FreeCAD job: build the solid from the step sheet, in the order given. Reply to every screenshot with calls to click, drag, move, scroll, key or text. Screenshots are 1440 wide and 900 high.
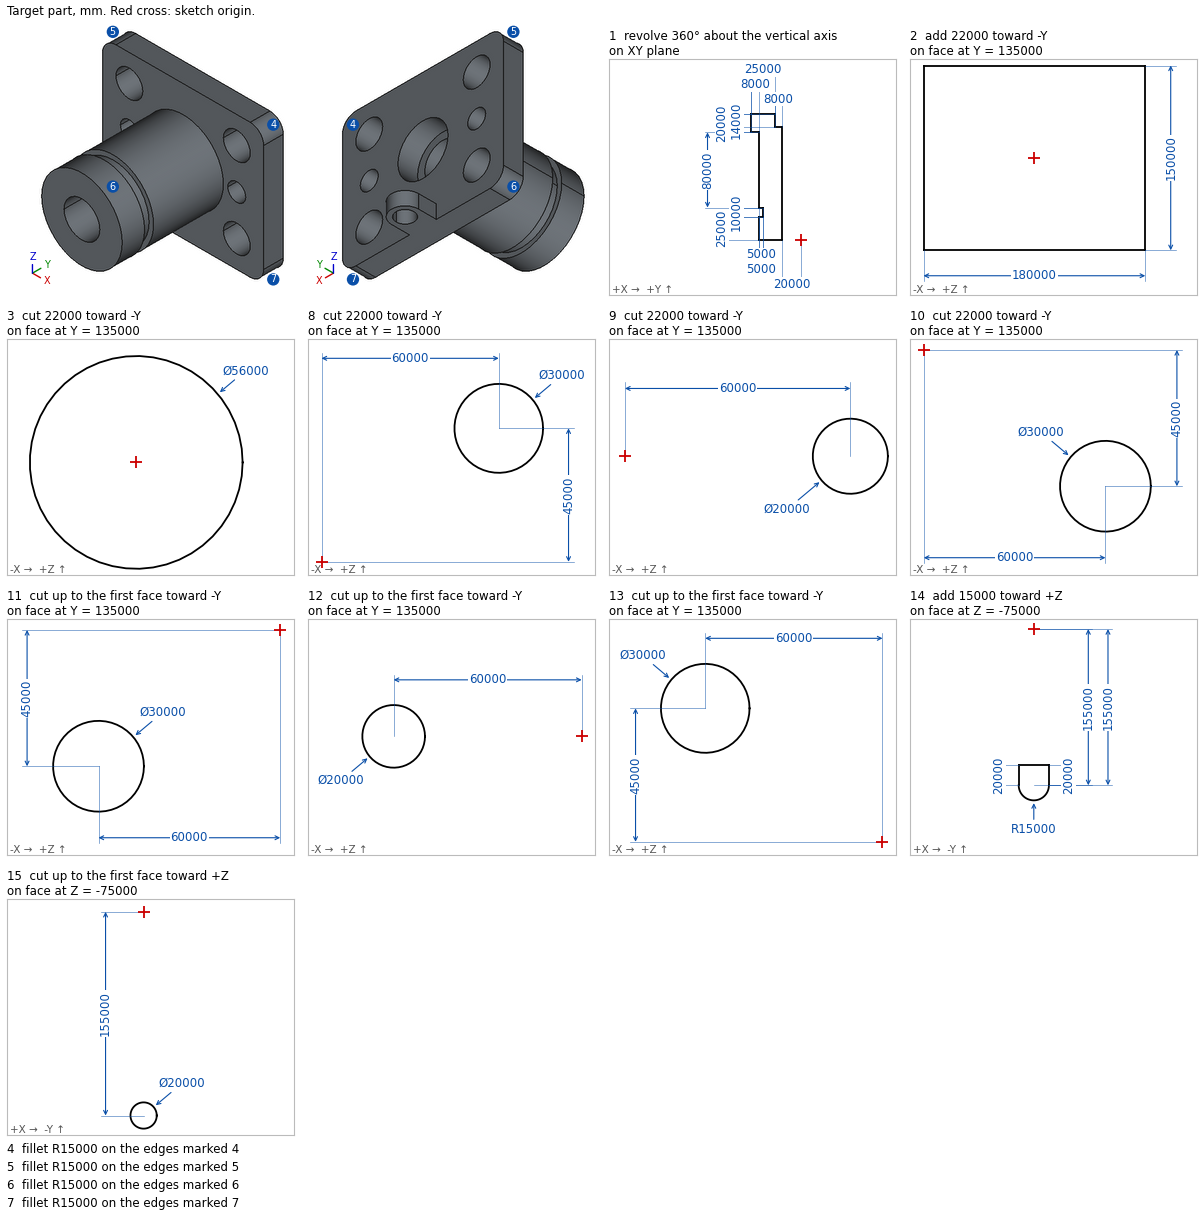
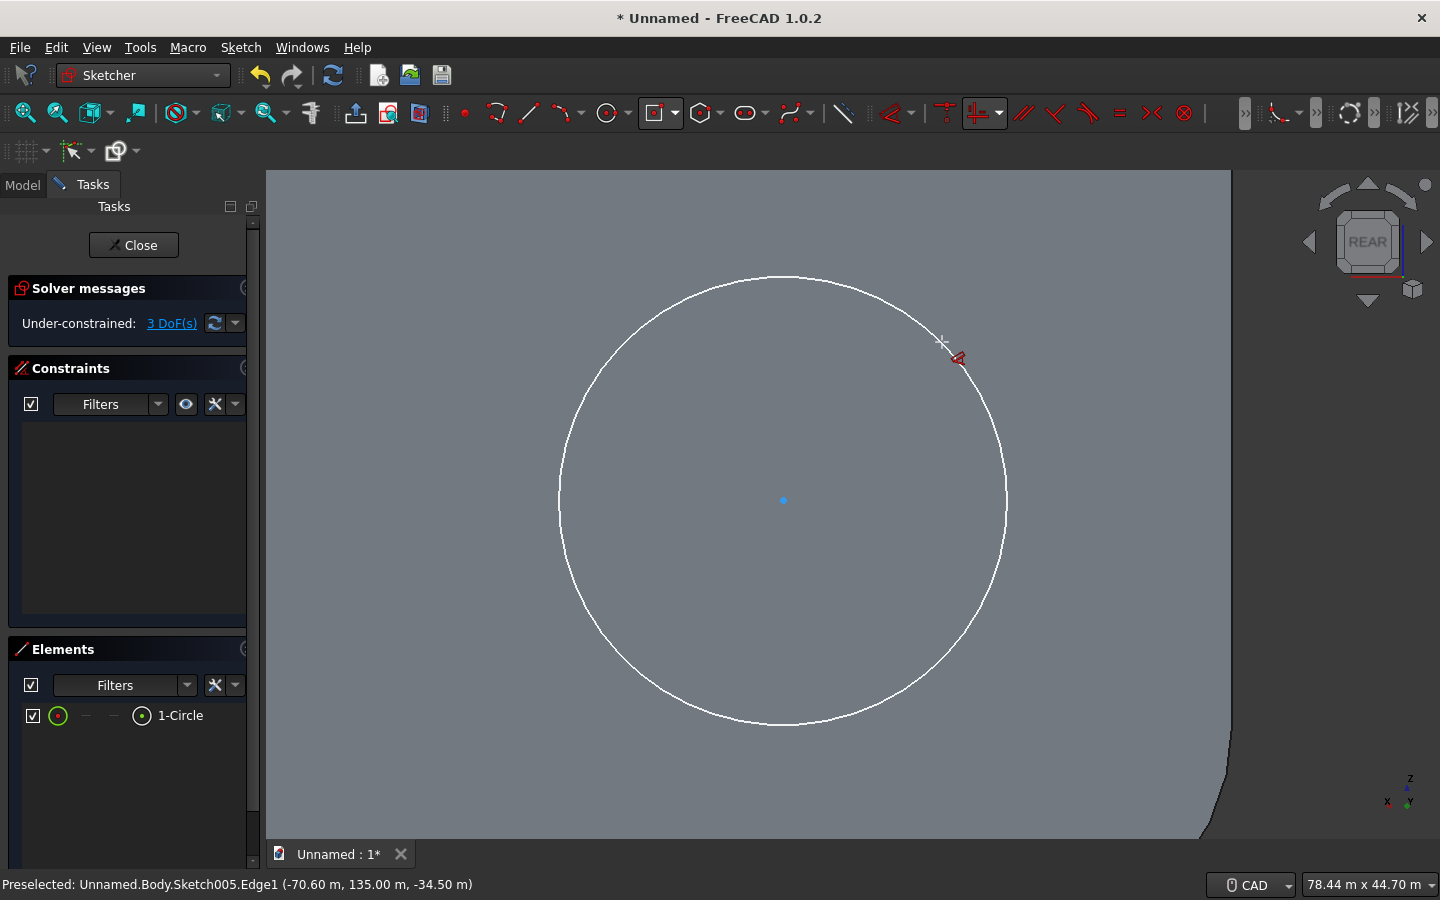
click(941, 342)
click(964, 319)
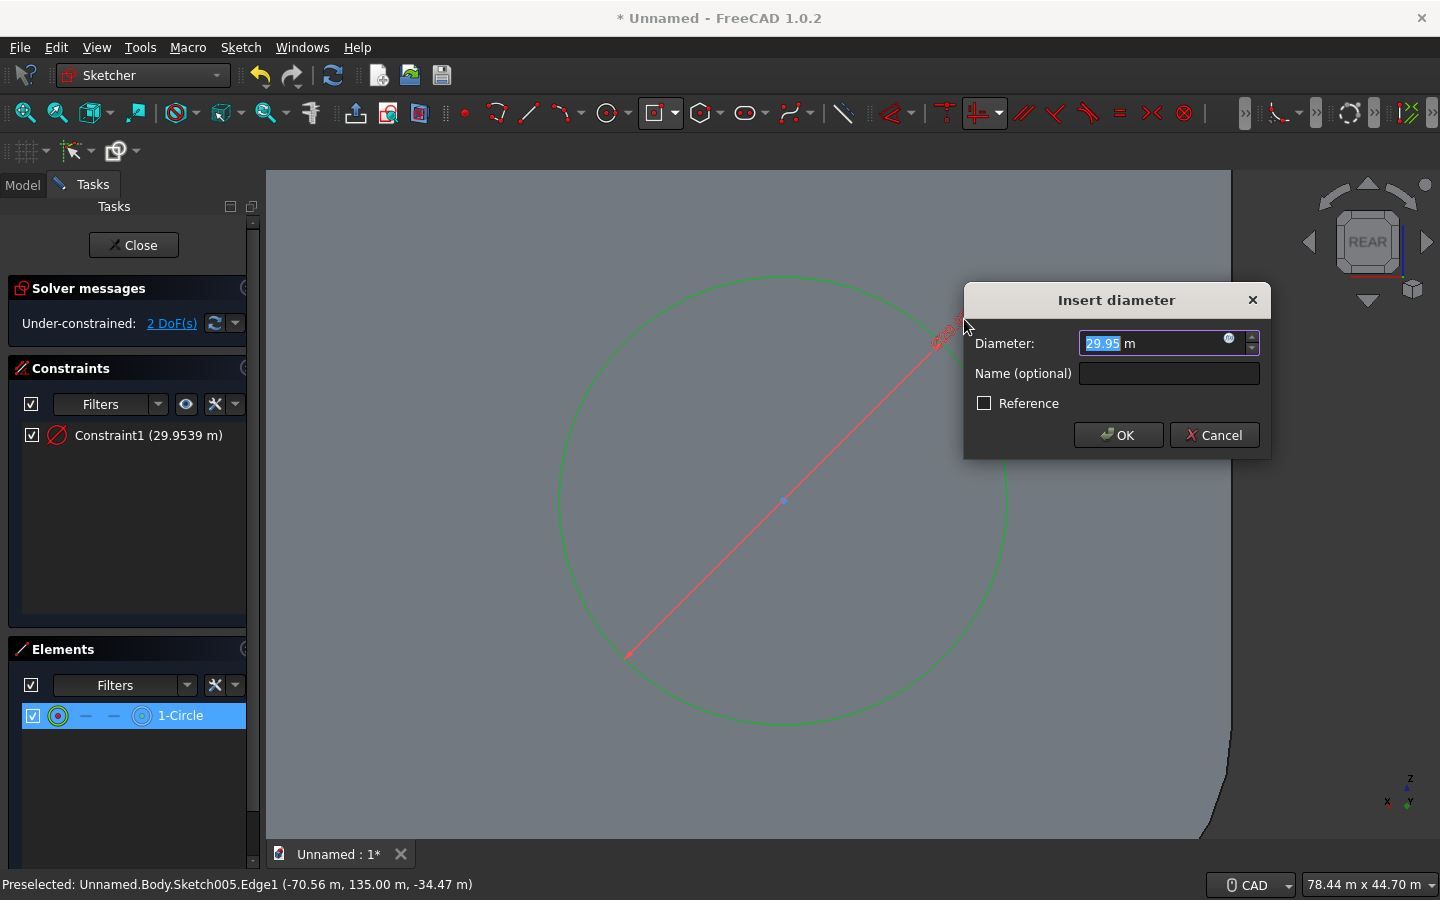
key(ctrl+a)
text(30000 mm)
key(Return)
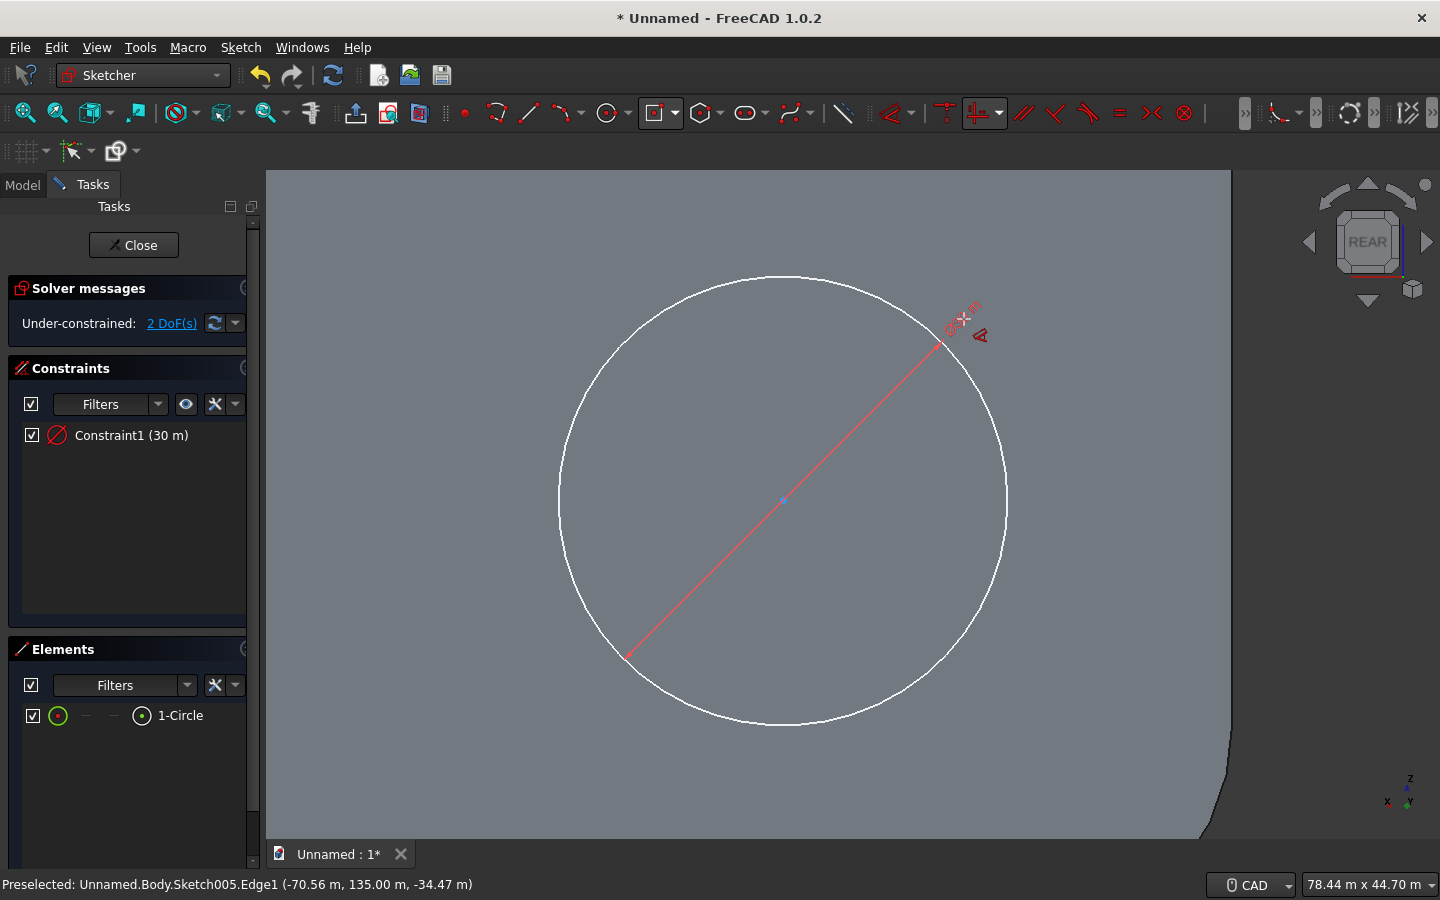
click(783, 501)
click(538, 535)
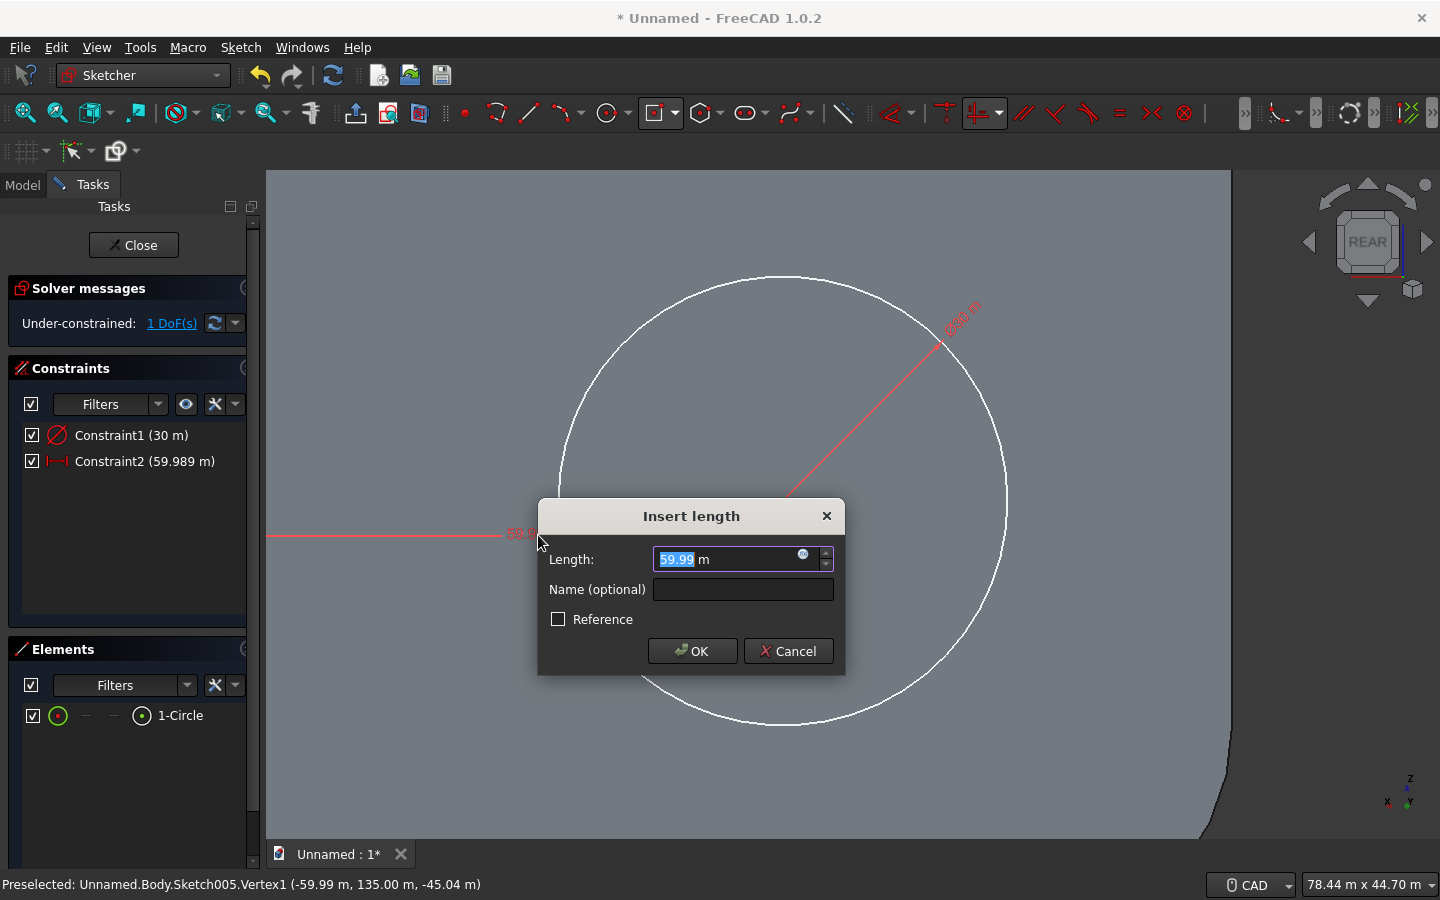
key(ctrl+a)
text(60000 mm)
key(Return)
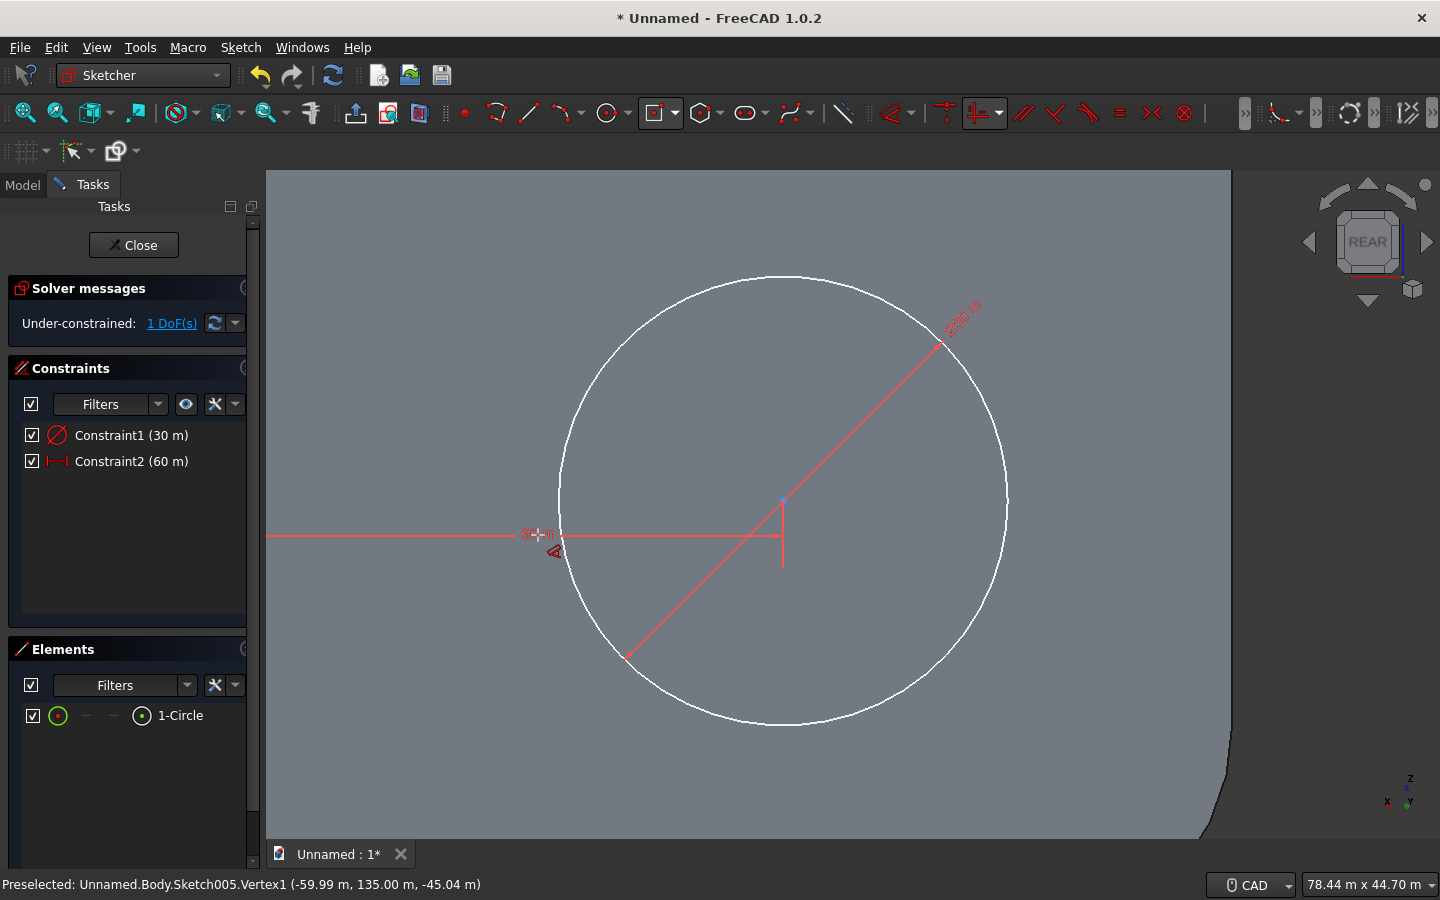
click(783, 501)
click(817, 349)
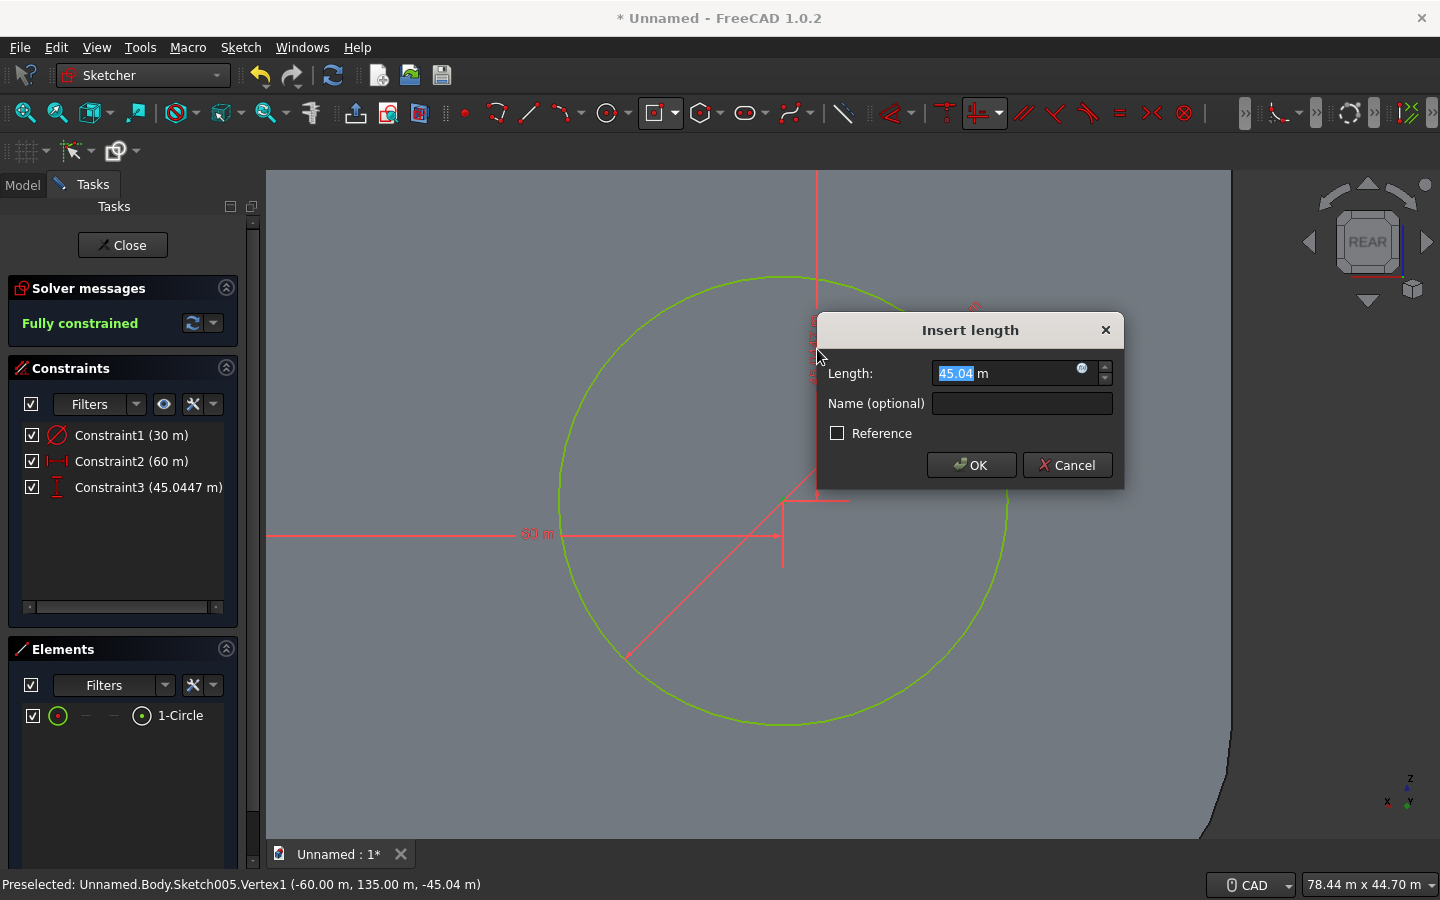
key(ctrl+a)
text(45000 mm)
key(Return)
key(Escape)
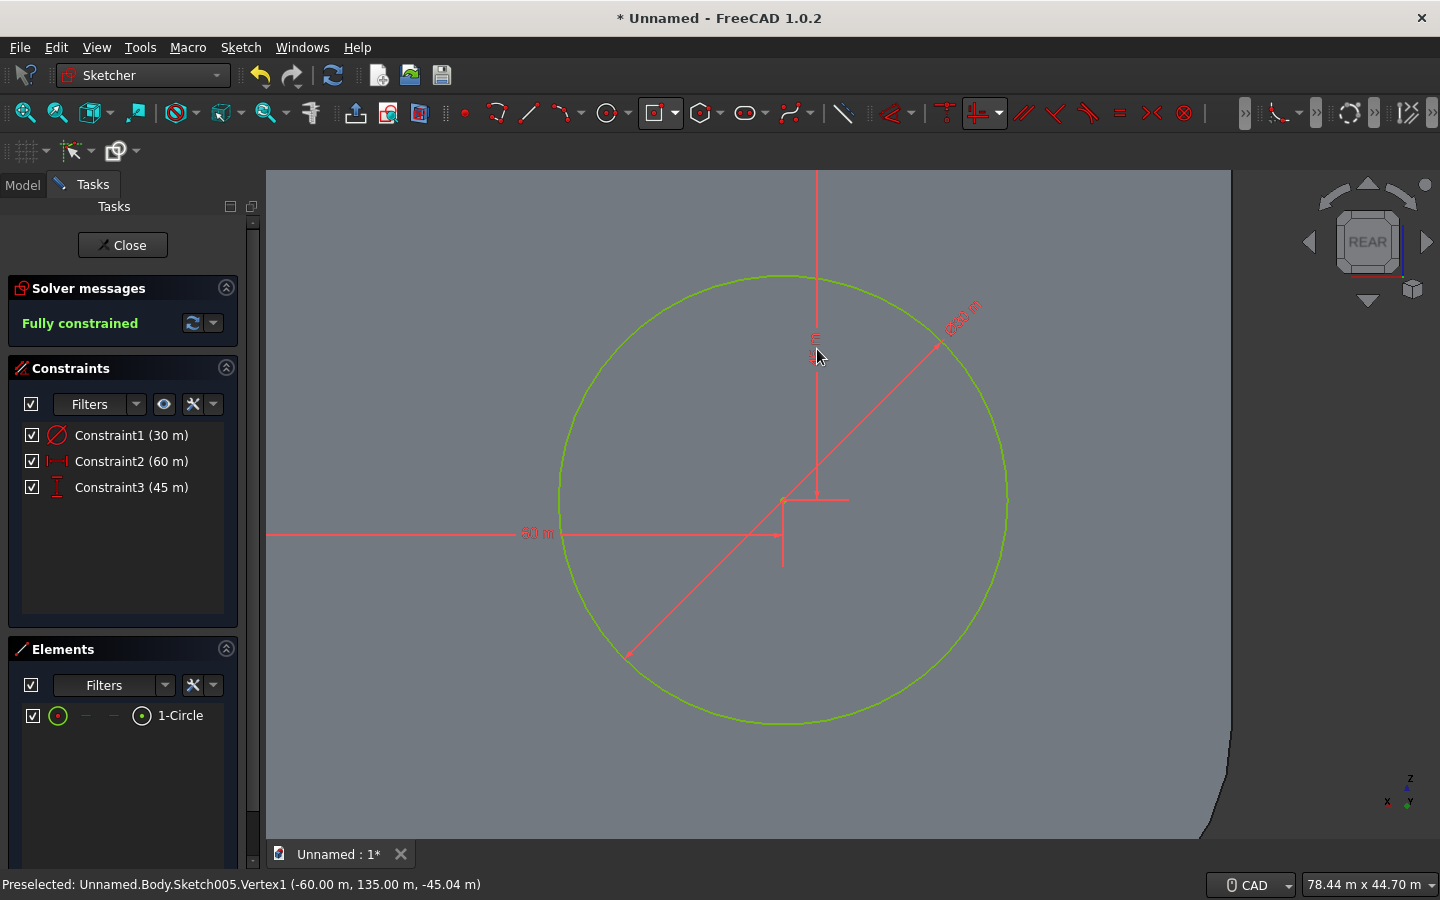
click(123, 245)